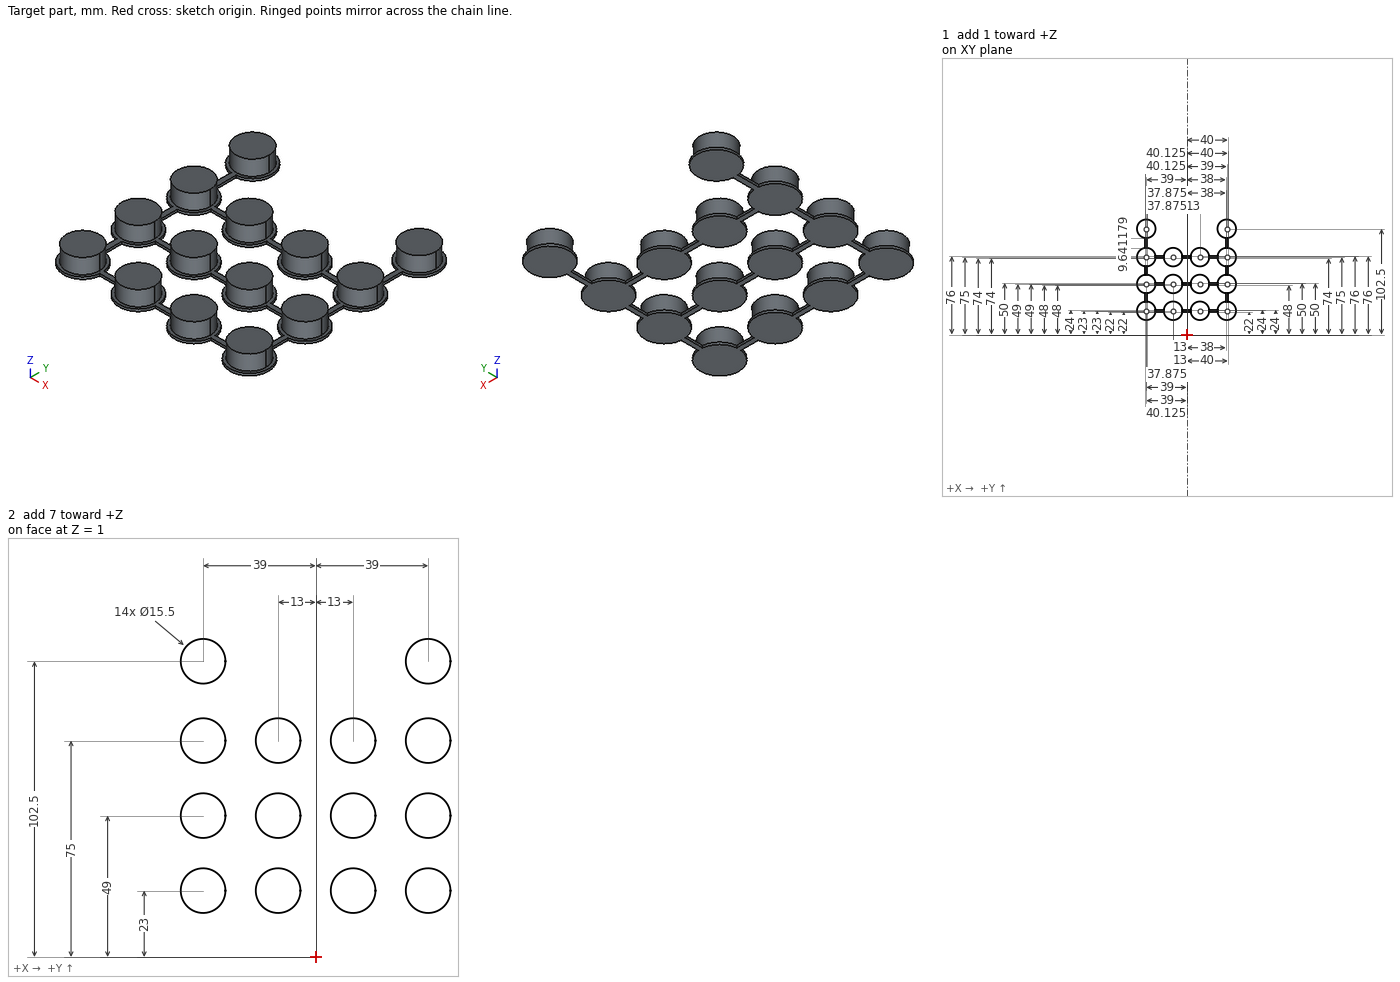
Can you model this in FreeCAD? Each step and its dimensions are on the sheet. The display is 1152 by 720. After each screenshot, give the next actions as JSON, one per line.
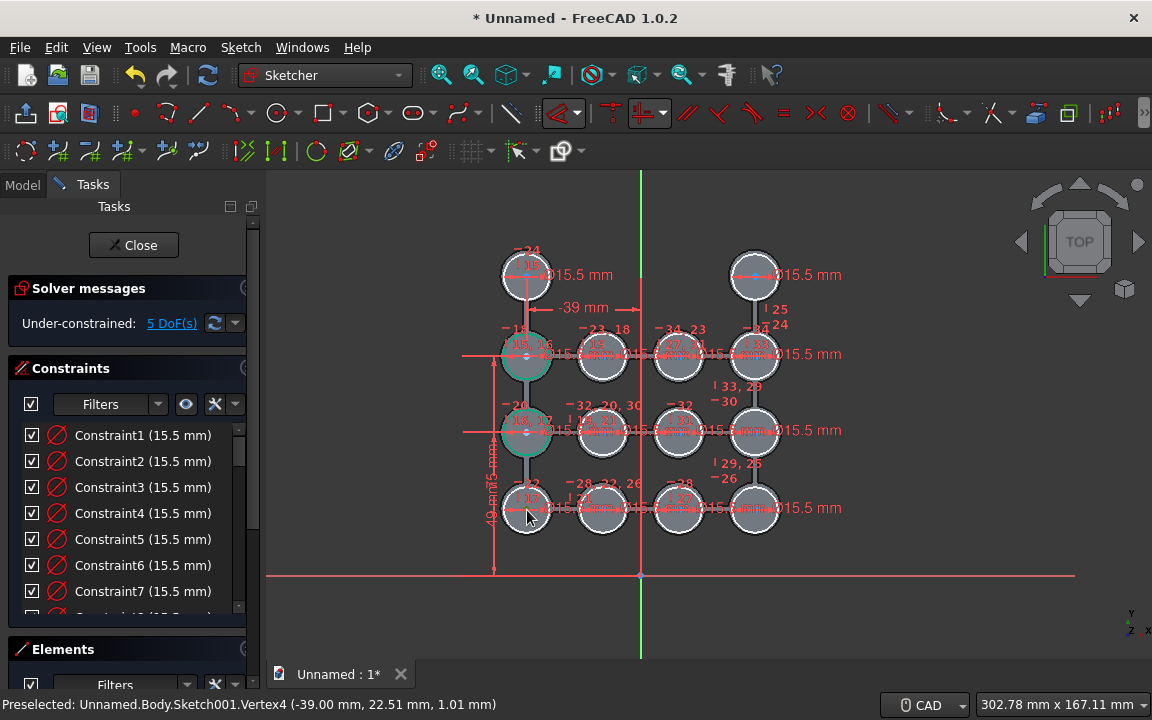
{"action": "key", "text": "i"}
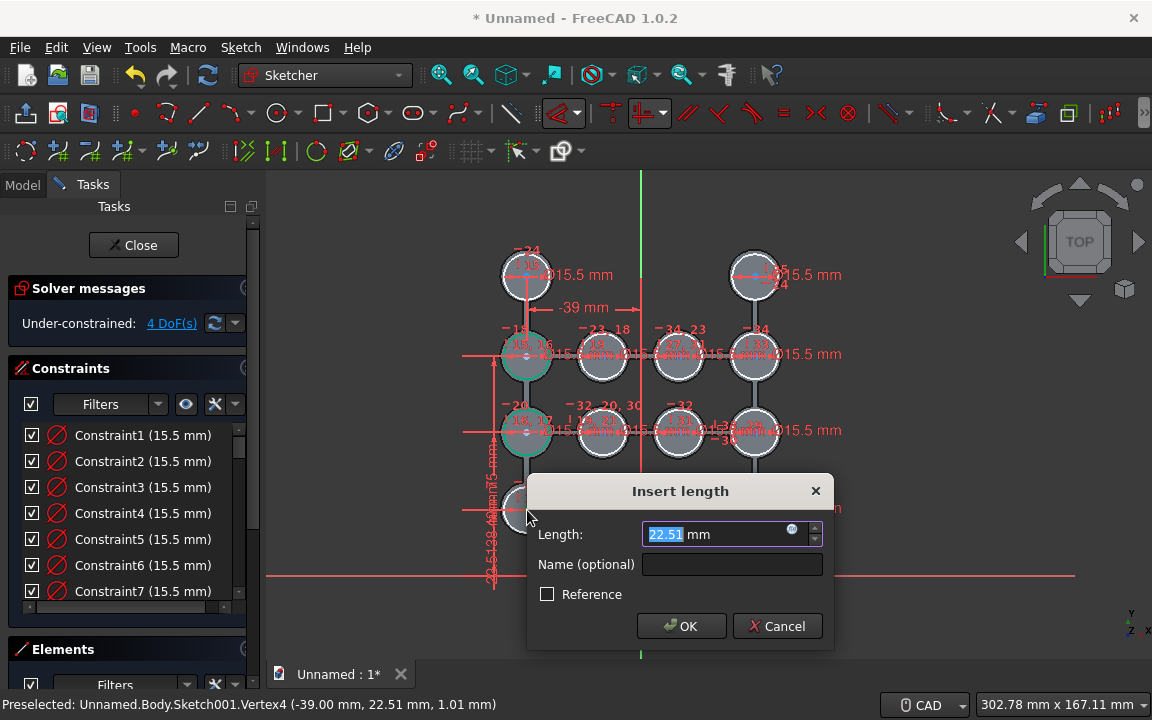
{"action": "type", "text": "23"}
{"action": "key", "text": "Return"}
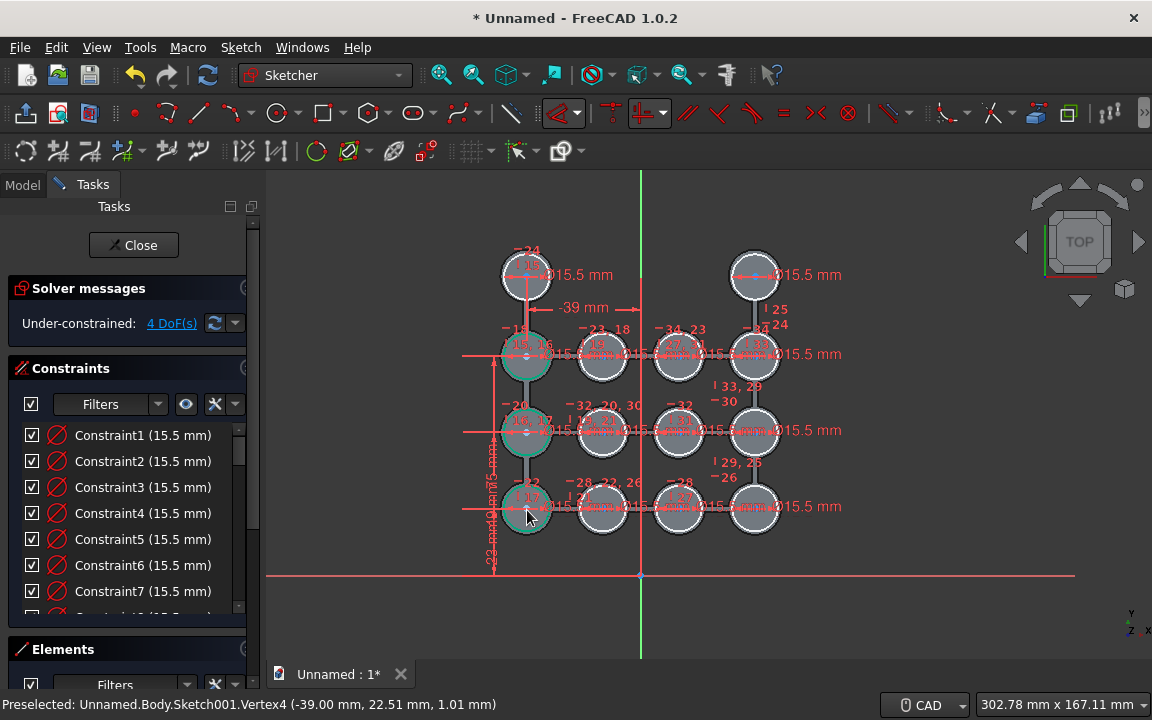
{"action": "left_click", "coordinate": [603, 356]}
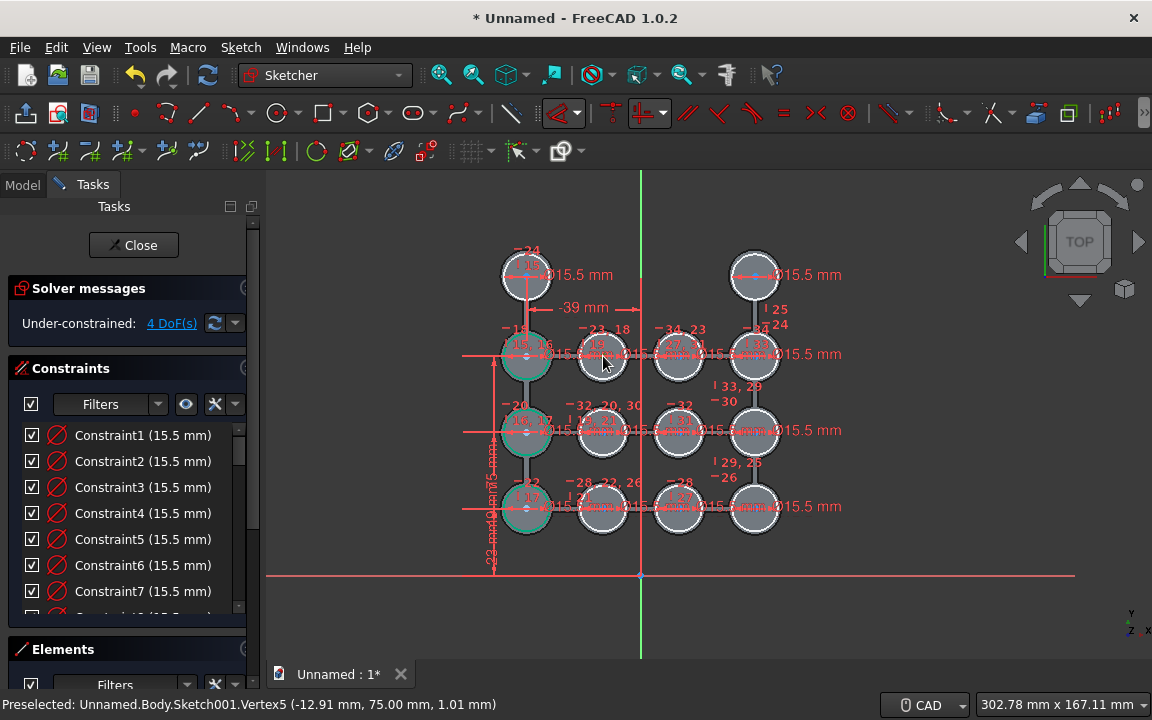
{"action": "left_click", "coordinate": [580, 114]}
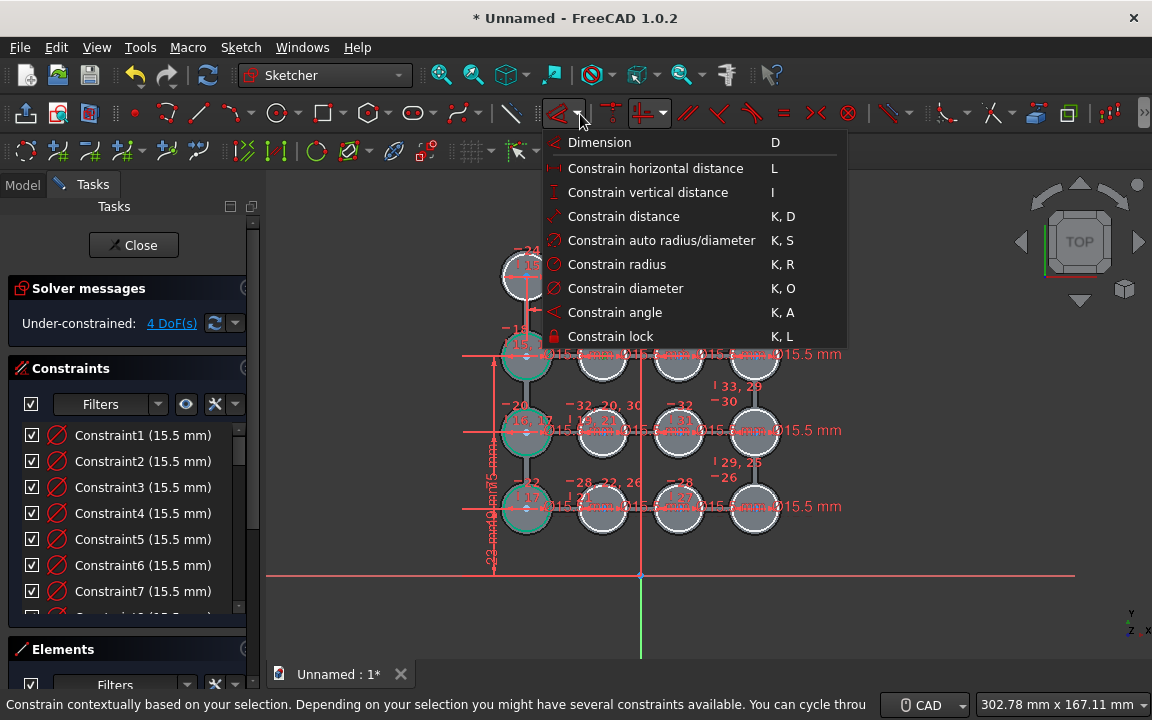
{"action": "left_click", "coordinate": [695, 168]}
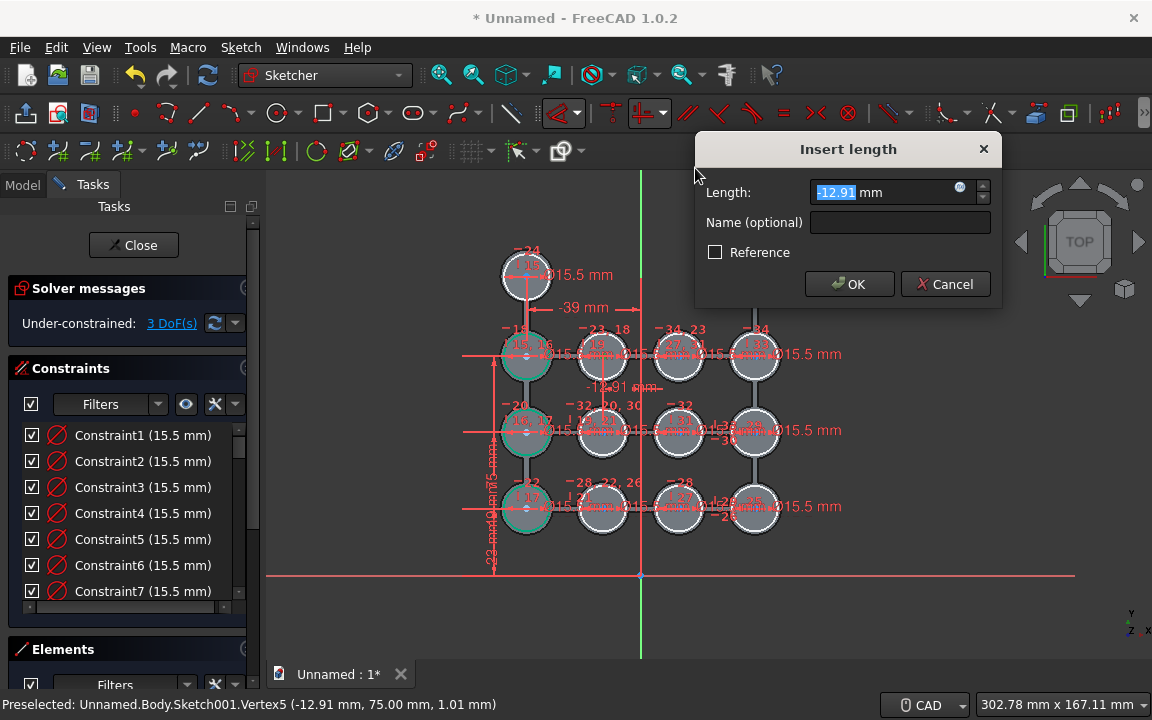
{"action": "type", "text": "-13"}
{"action": "key", "text": "Return"}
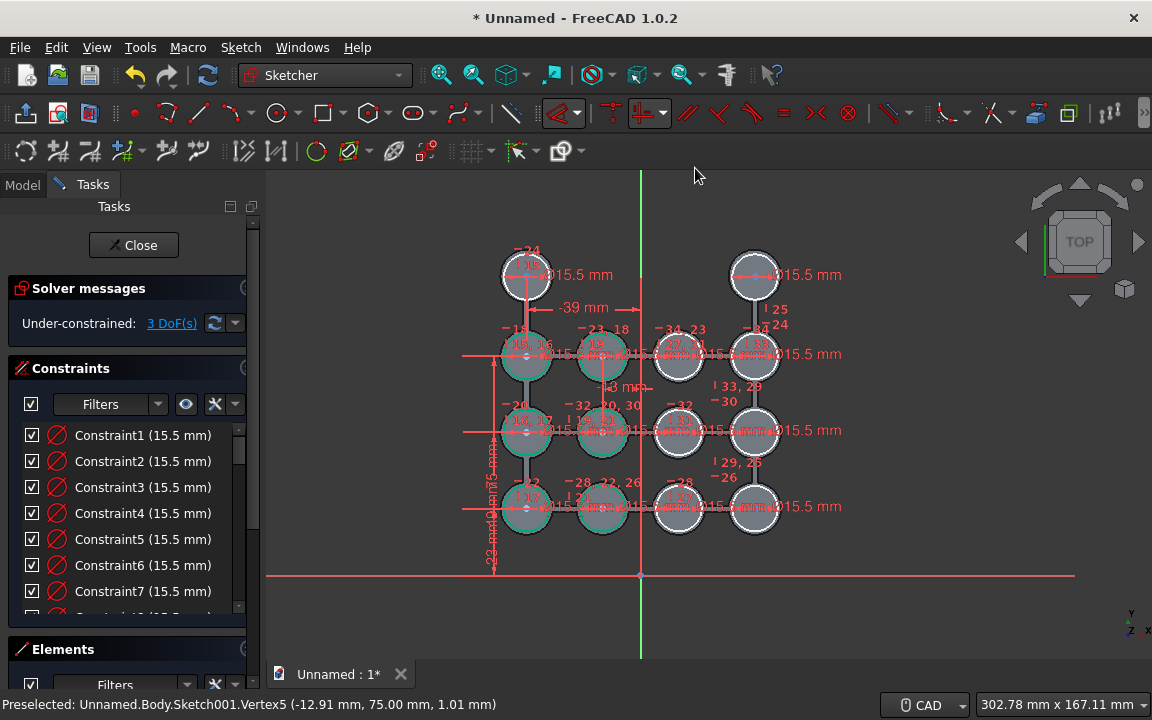
{"action": "left_click", "coordinate": [679, 356]}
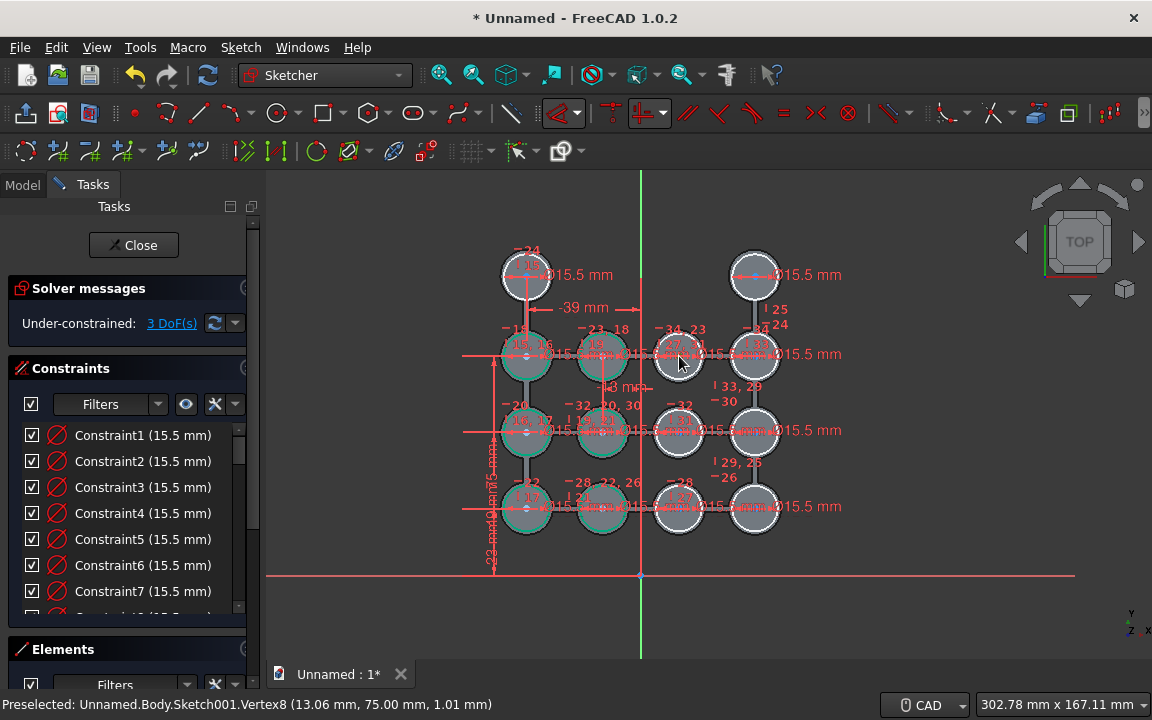
{"action": "key", "text": "l"}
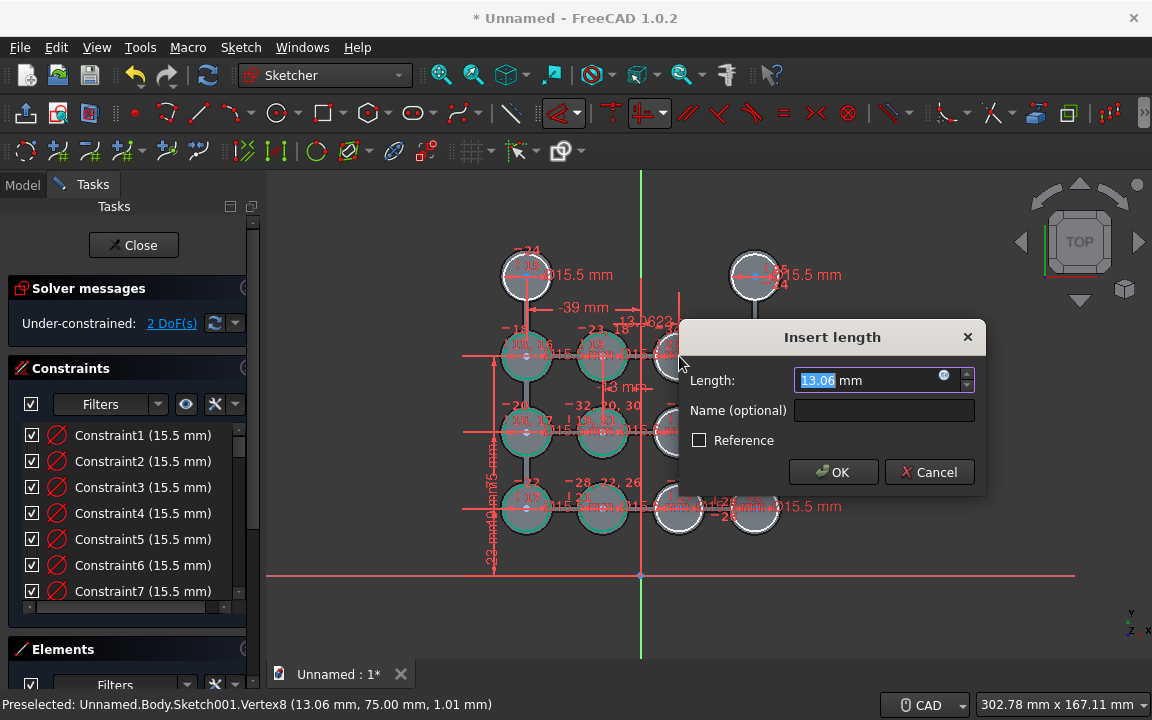
{"action": "type", "text": "13"}
{"action": "key", "text": "Return"}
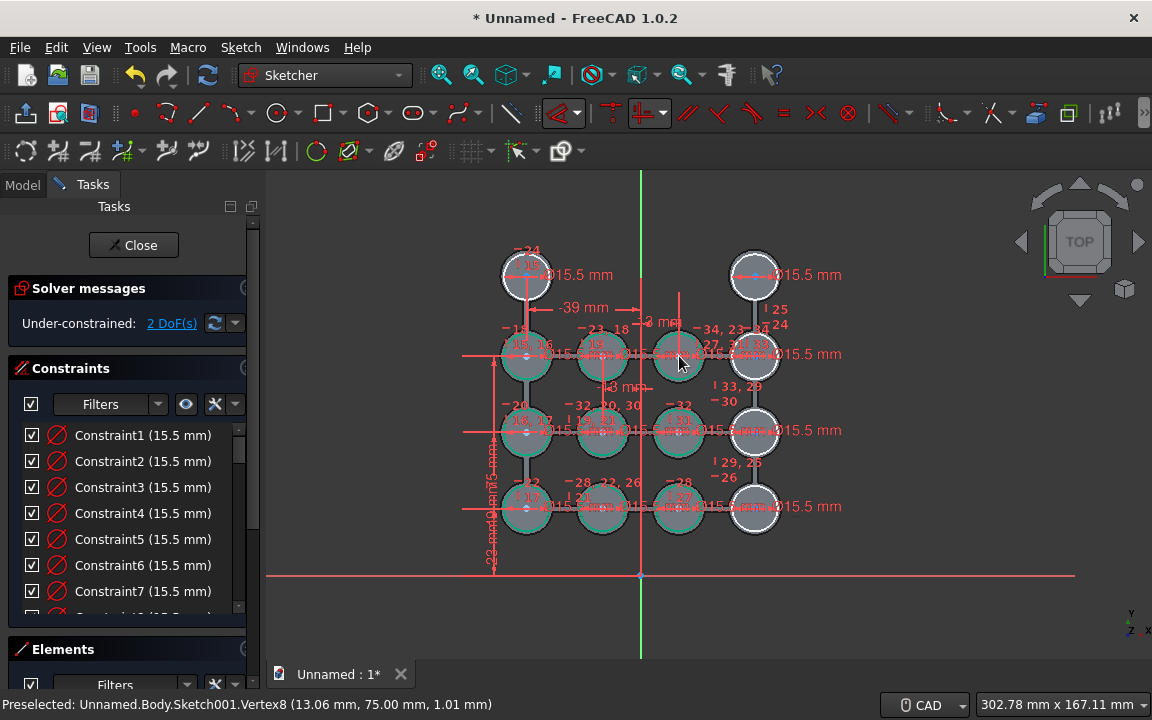
{"action": "left_click", "coordinate": [755, 277]}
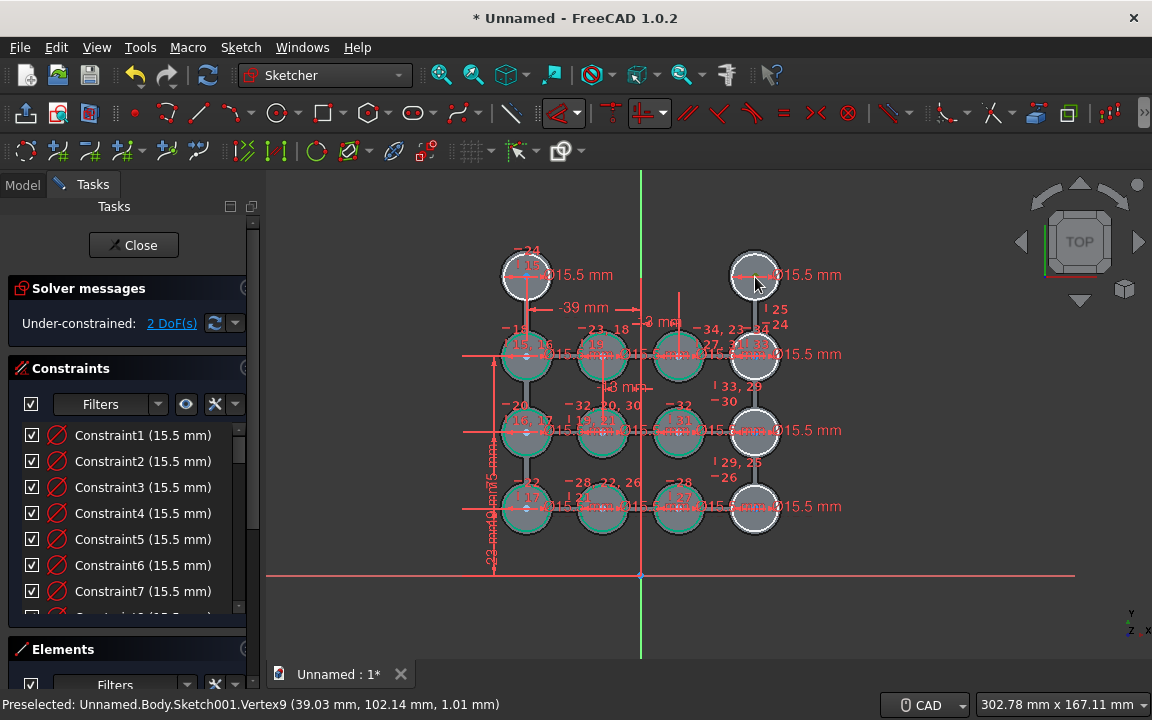
{"action": "left_click", "coordinate": [580, 114]}